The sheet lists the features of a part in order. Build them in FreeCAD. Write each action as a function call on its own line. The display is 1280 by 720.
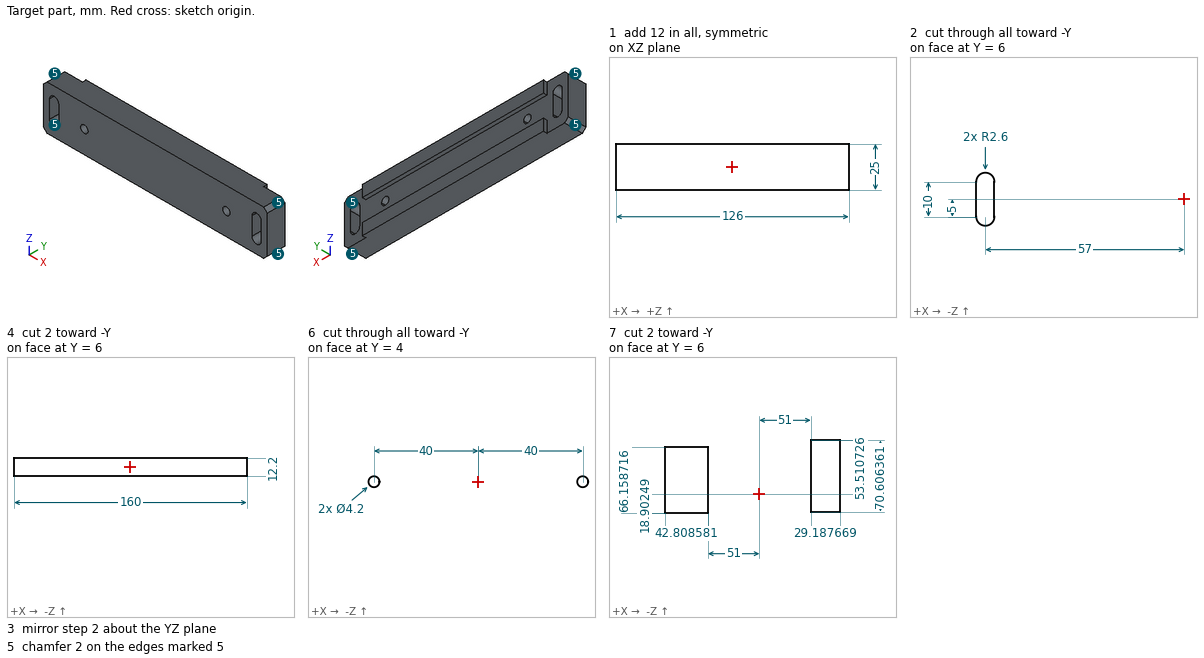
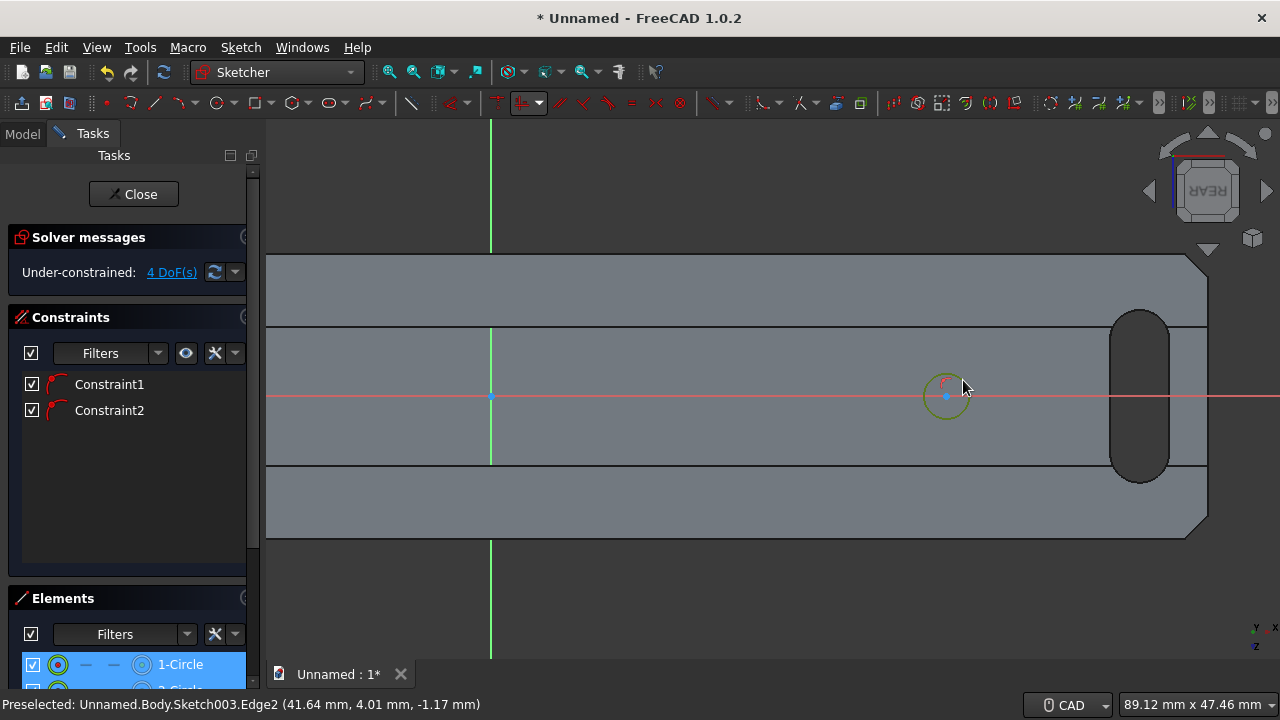
click(632, 104)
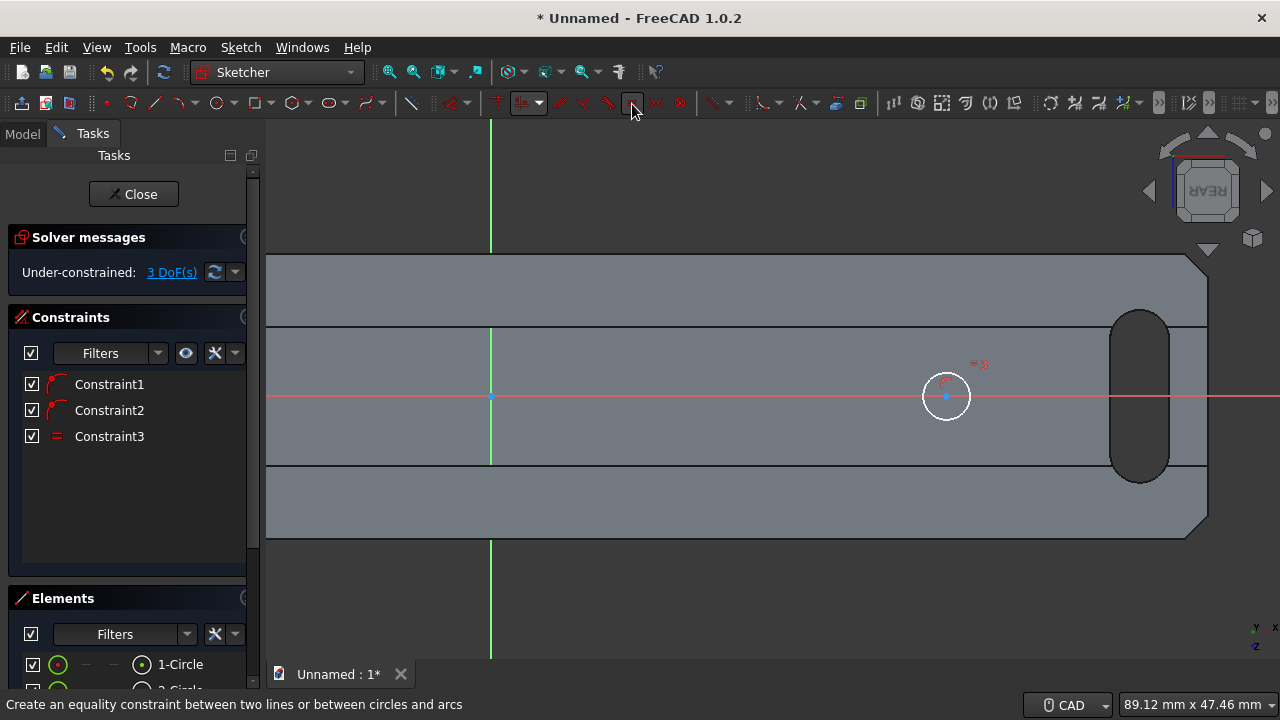
click(450, 104)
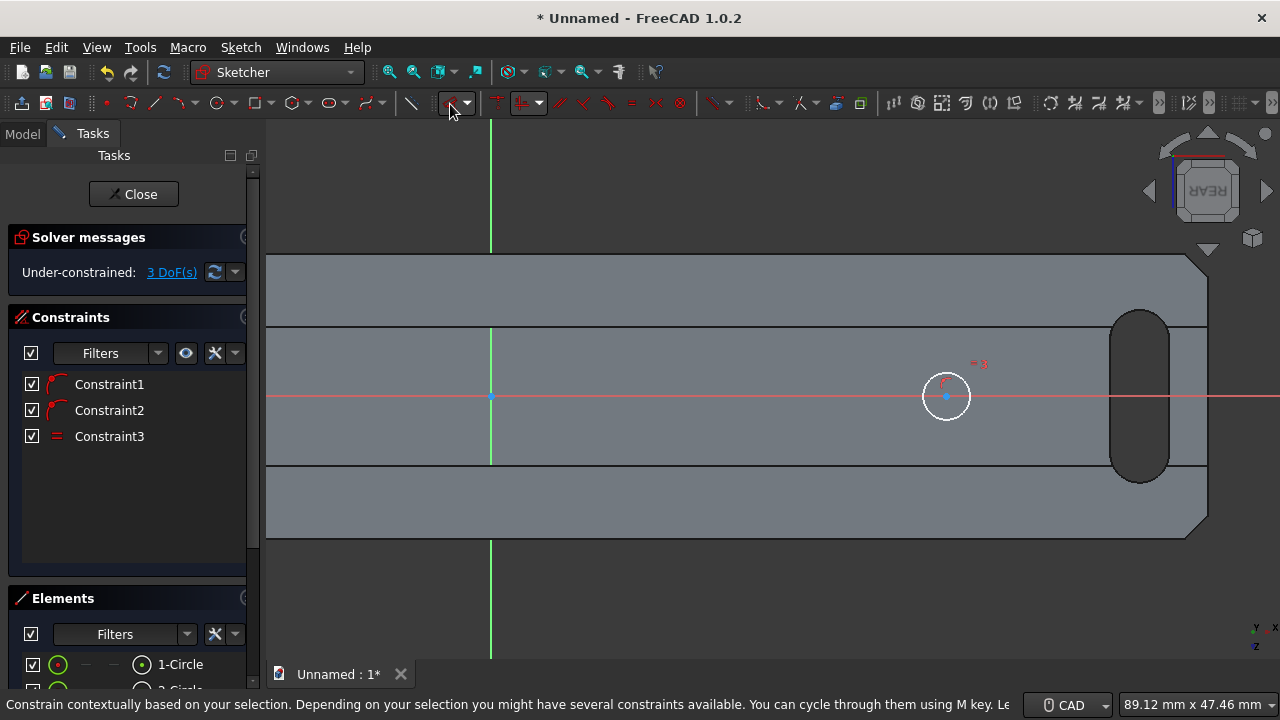
scroll(964, 380, down, 3)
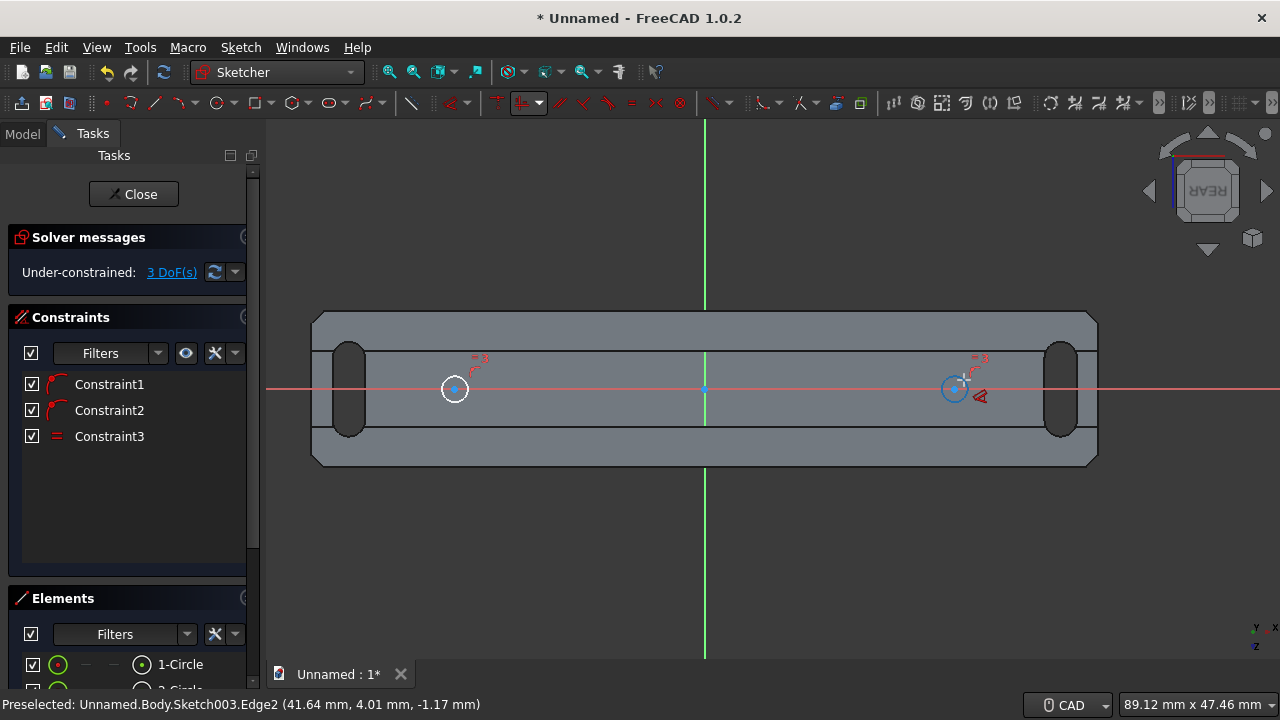
scroll(464, 380, up, 3)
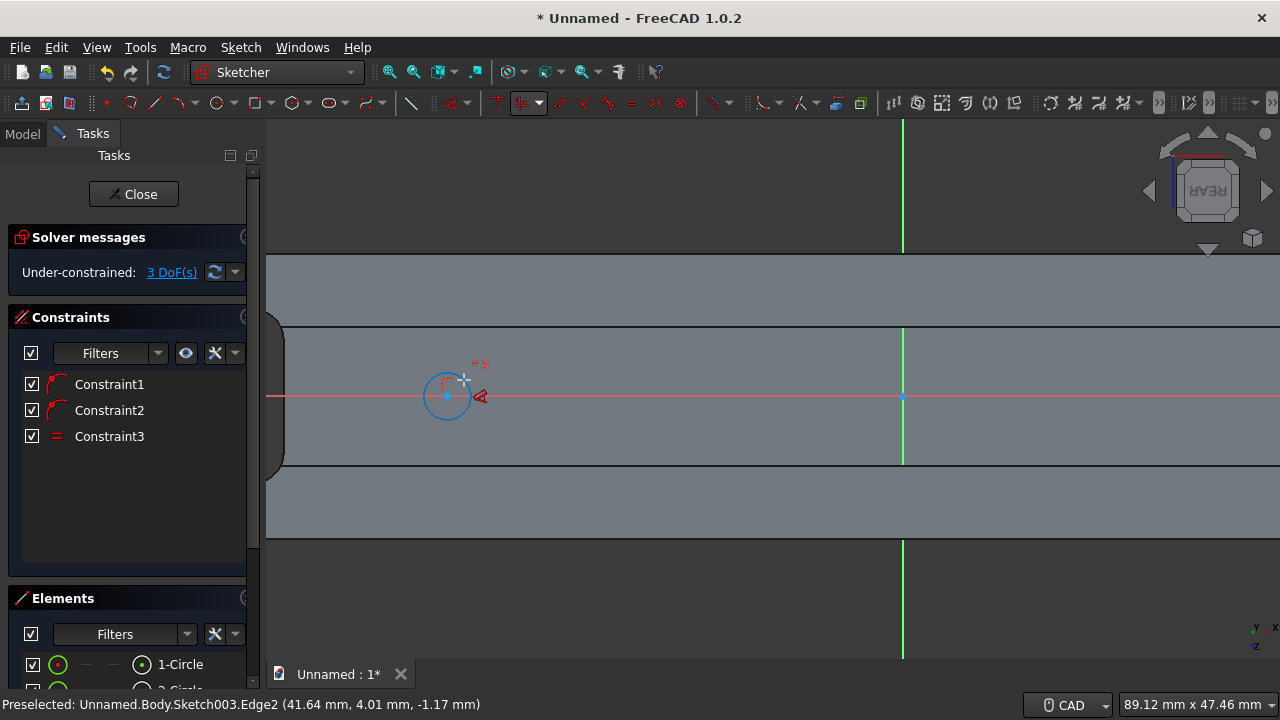
click(464, 380)
click(487, 358)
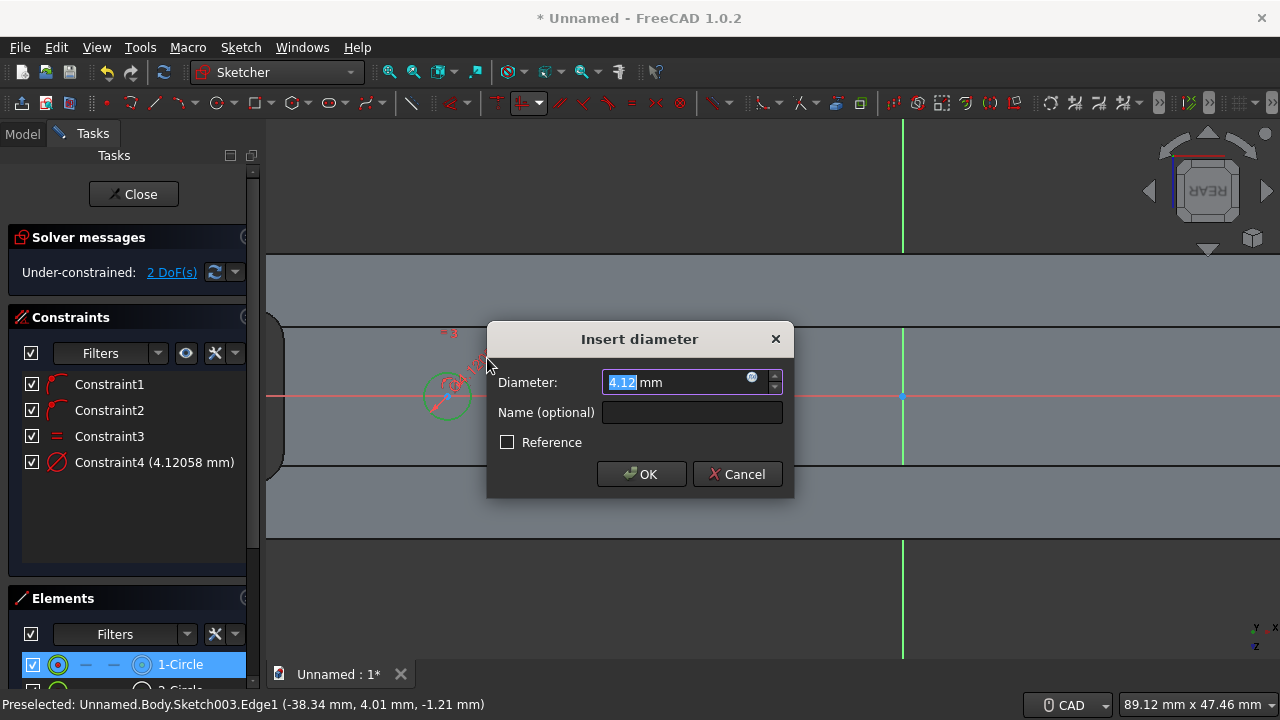
text(4.2)
key(Return)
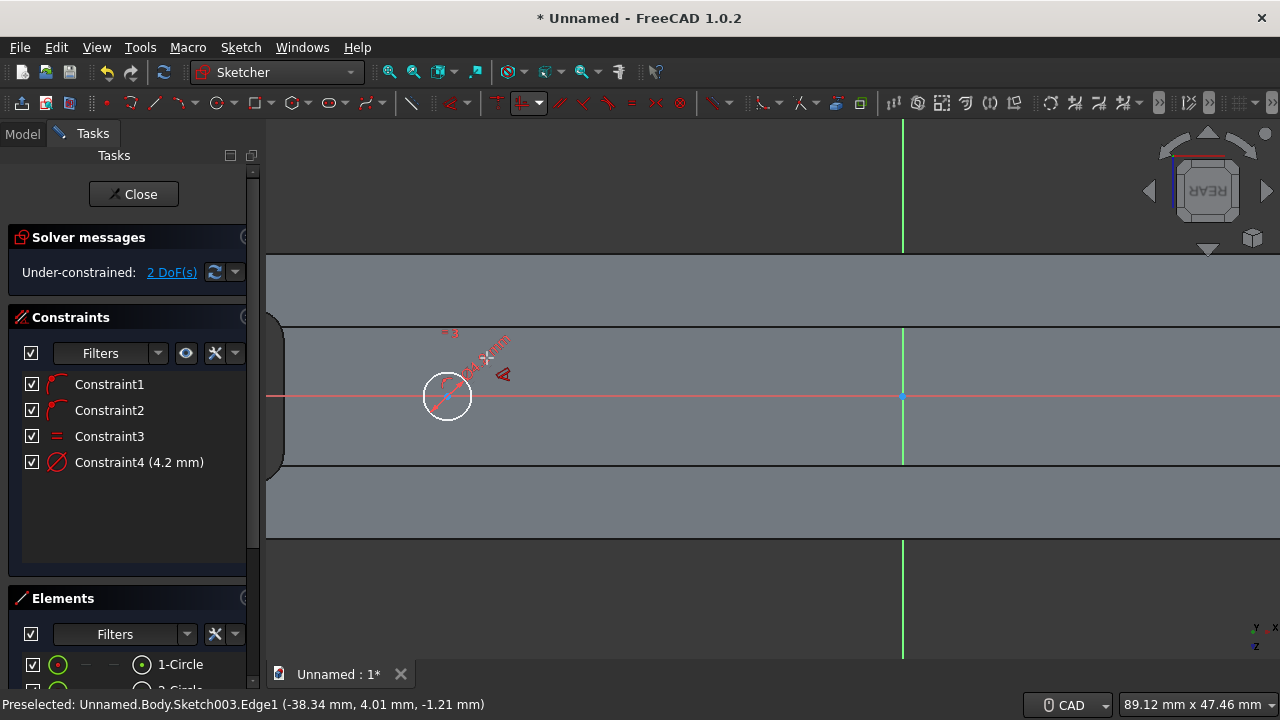
click(447, 396)
click(675, 430)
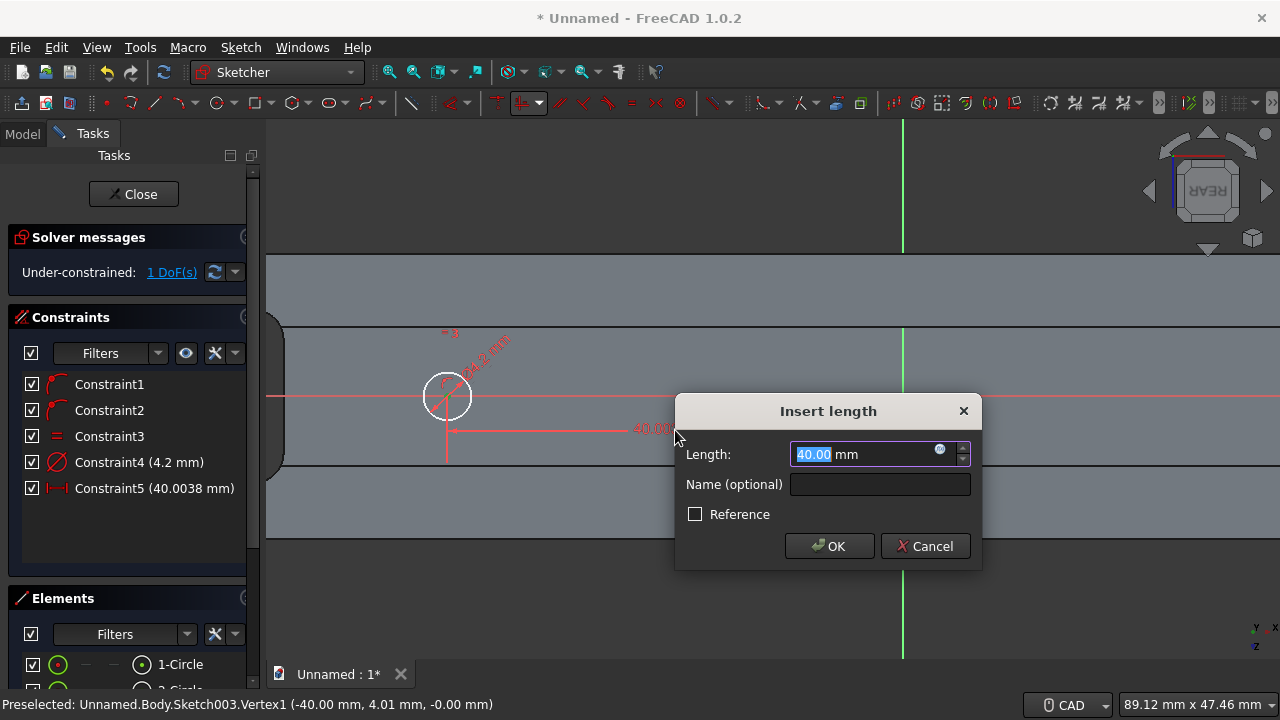
text(40)
key(Return)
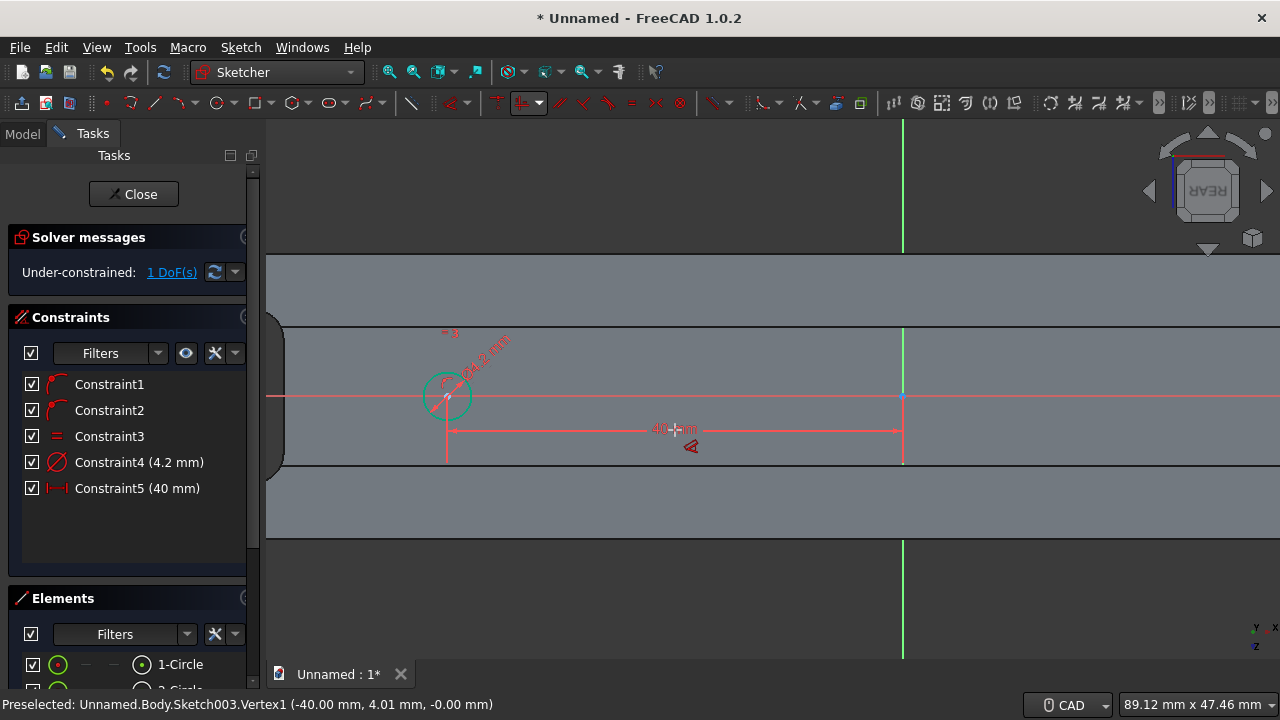
scroll(464, 380, down, 3)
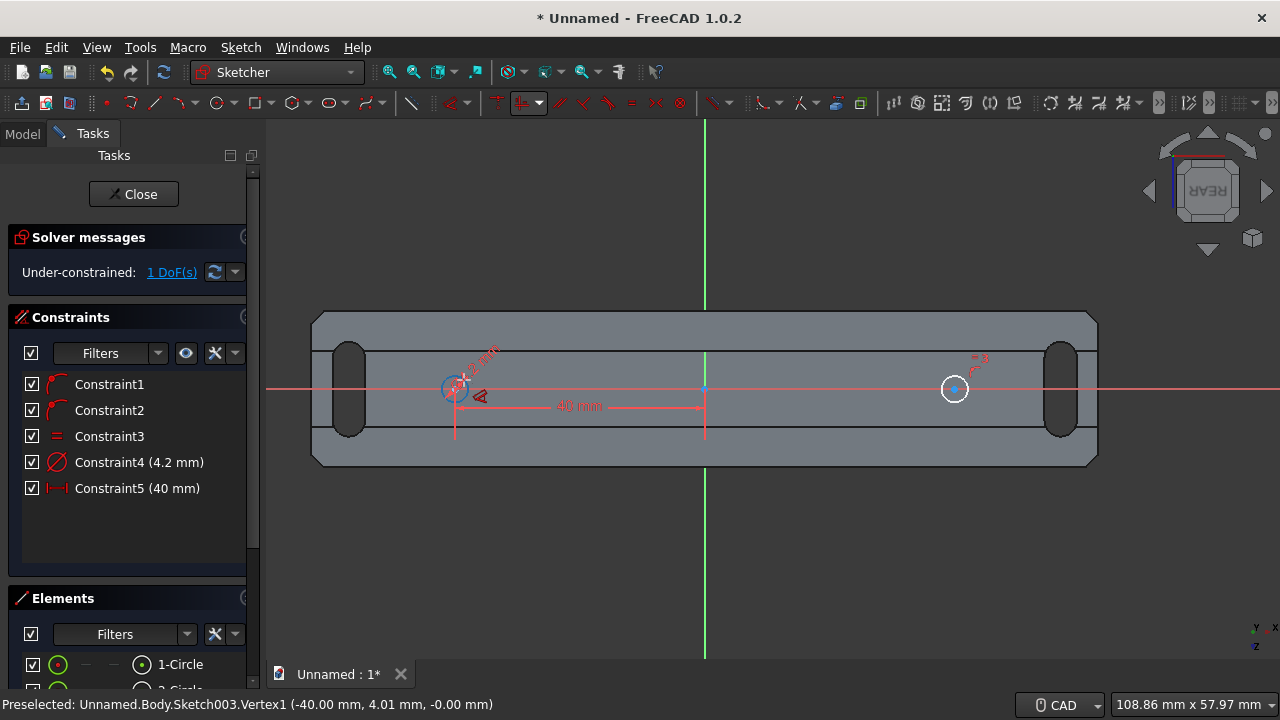
click(955, 389)
click(830, 423)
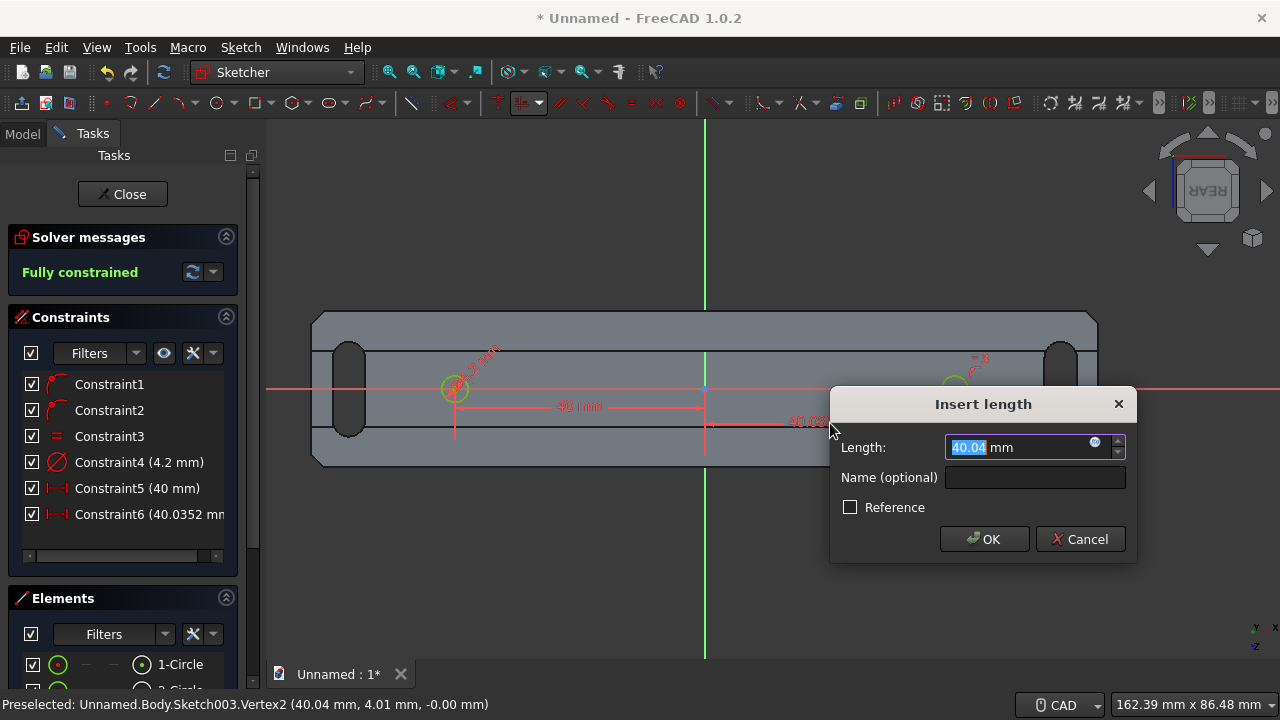
text(40)
key(Return)
key(Escape)